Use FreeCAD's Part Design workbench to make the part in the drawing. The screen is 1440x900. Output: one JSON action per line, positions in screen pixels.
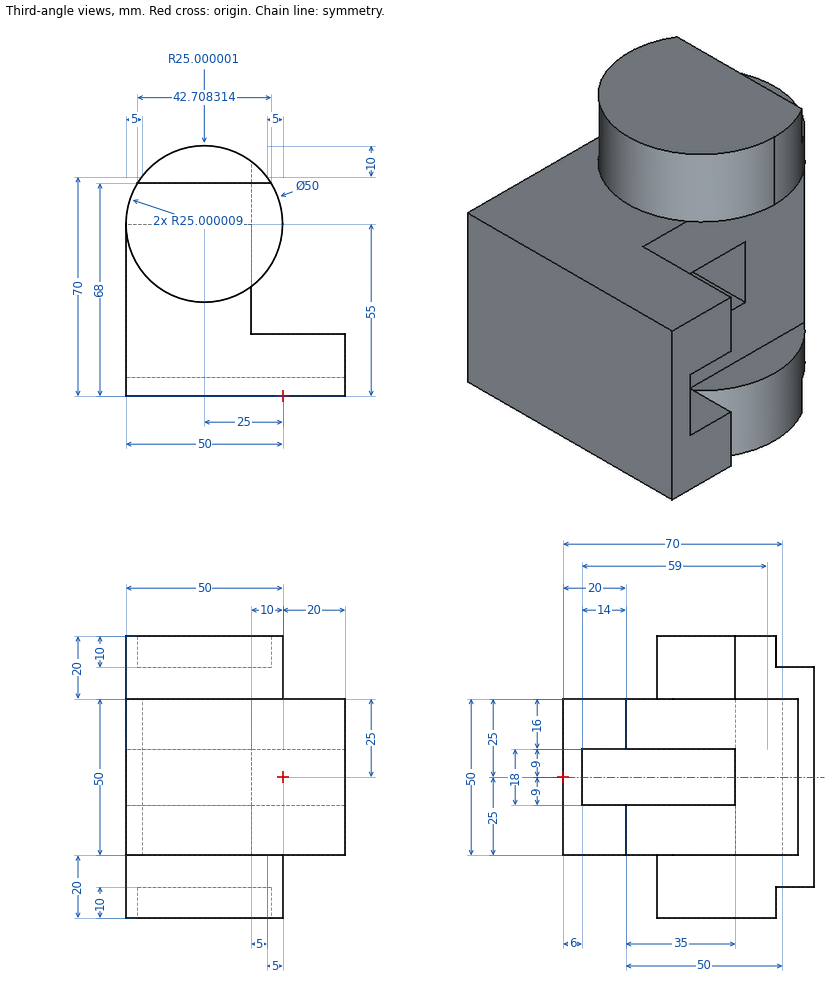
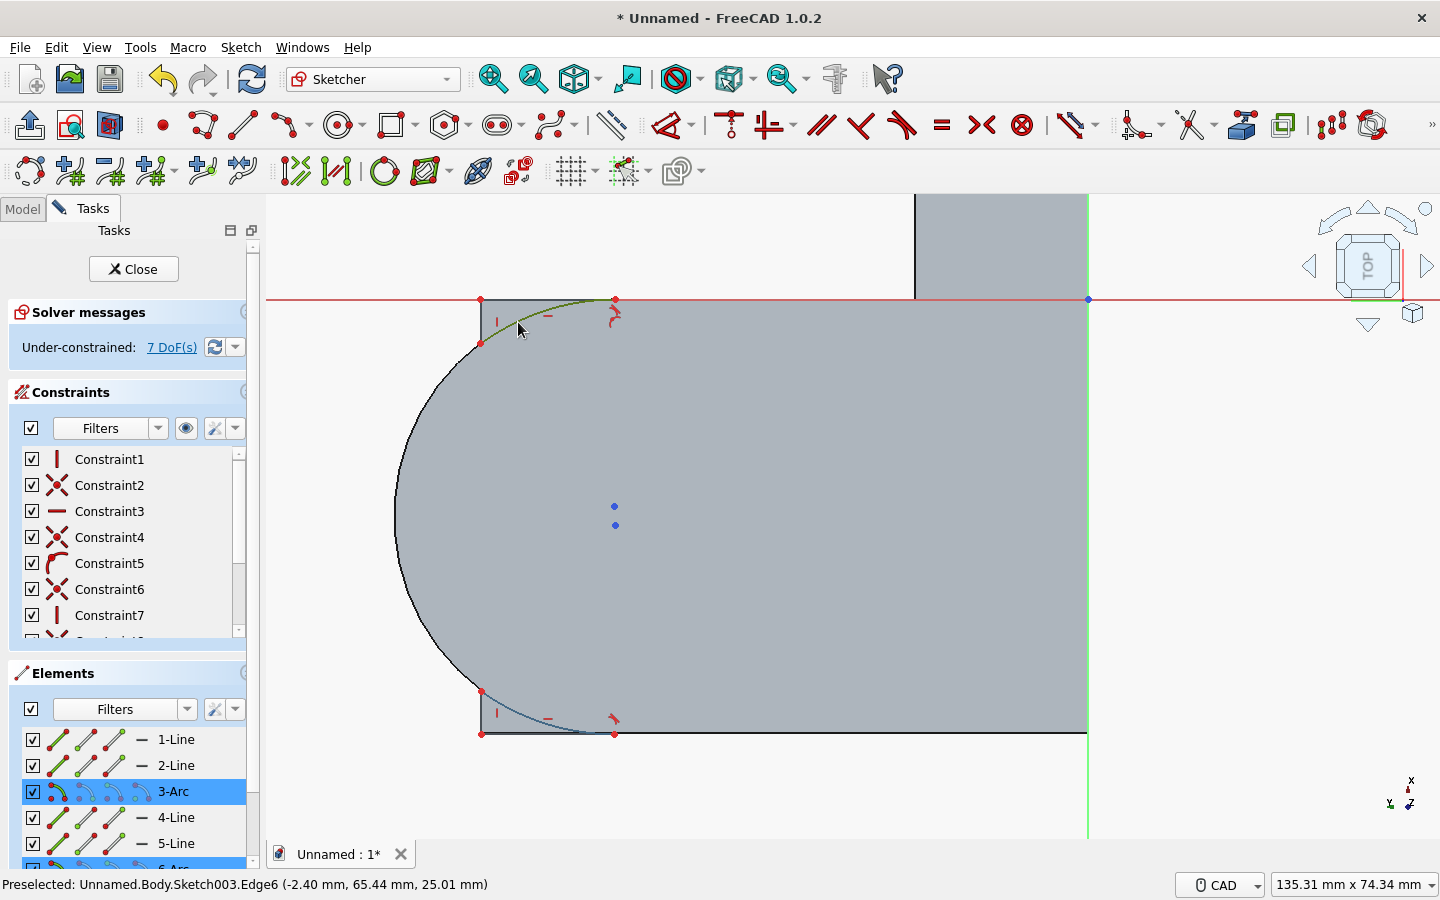
{"action": "left_click", "coordinate": [730, 126]}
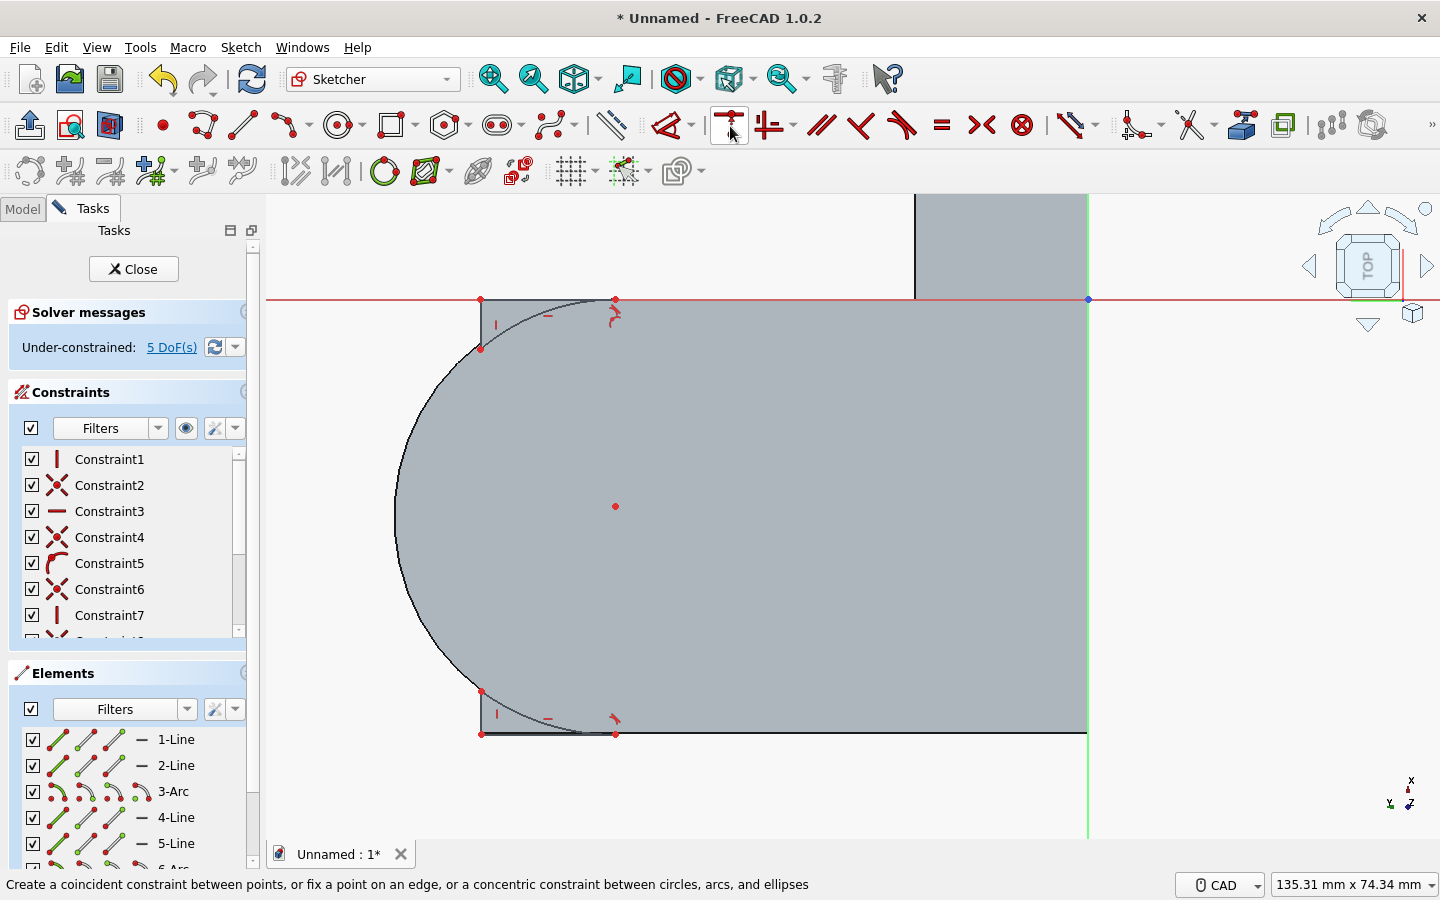
{"action": "left_click", "coordinate": [518, 713]}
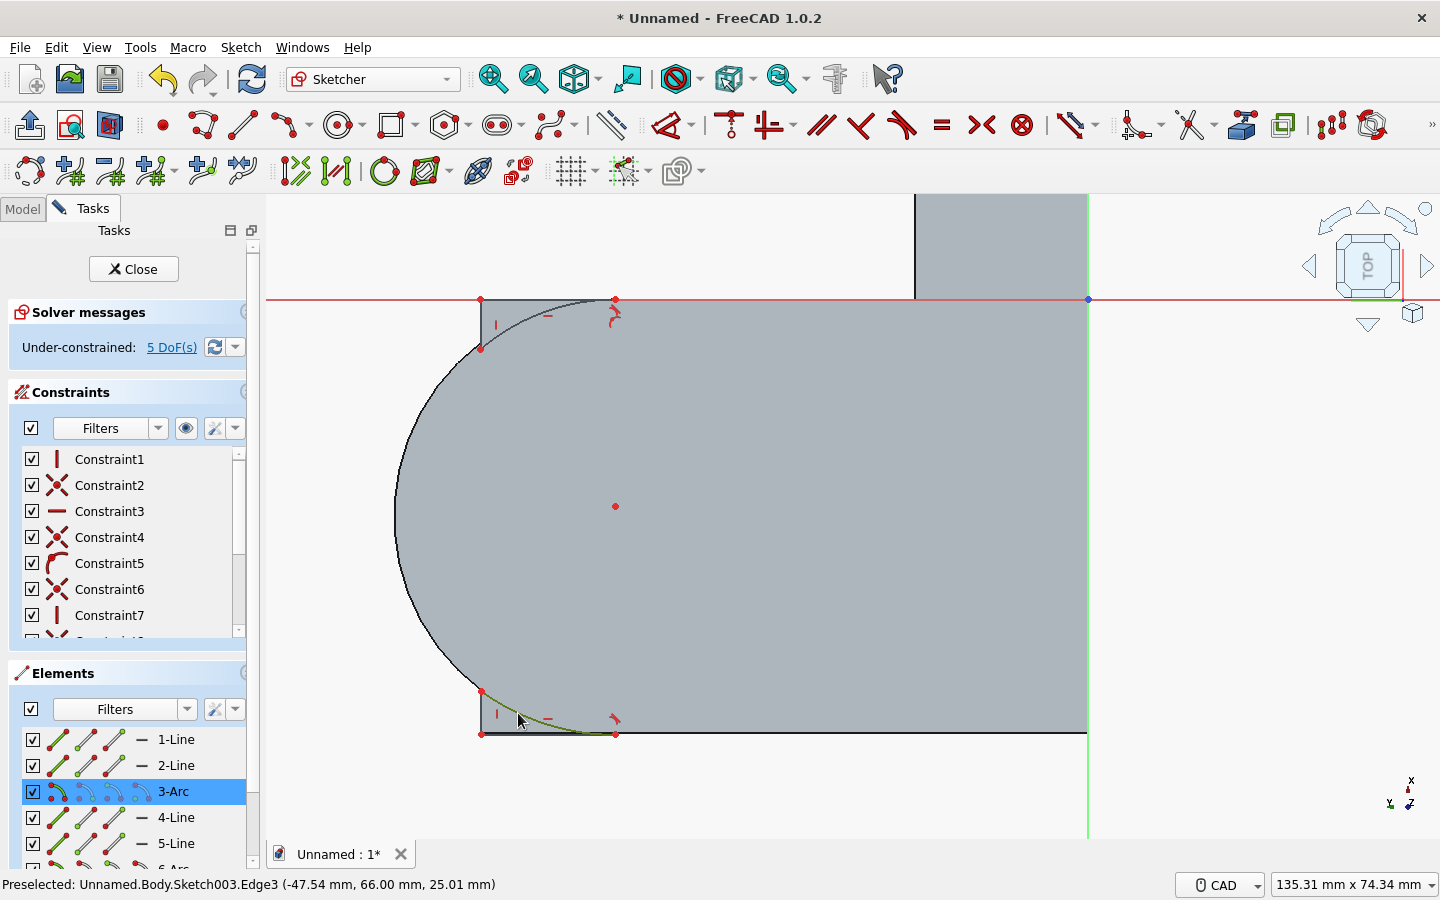
{"action": "left_click", "coordinate": [517, 324]}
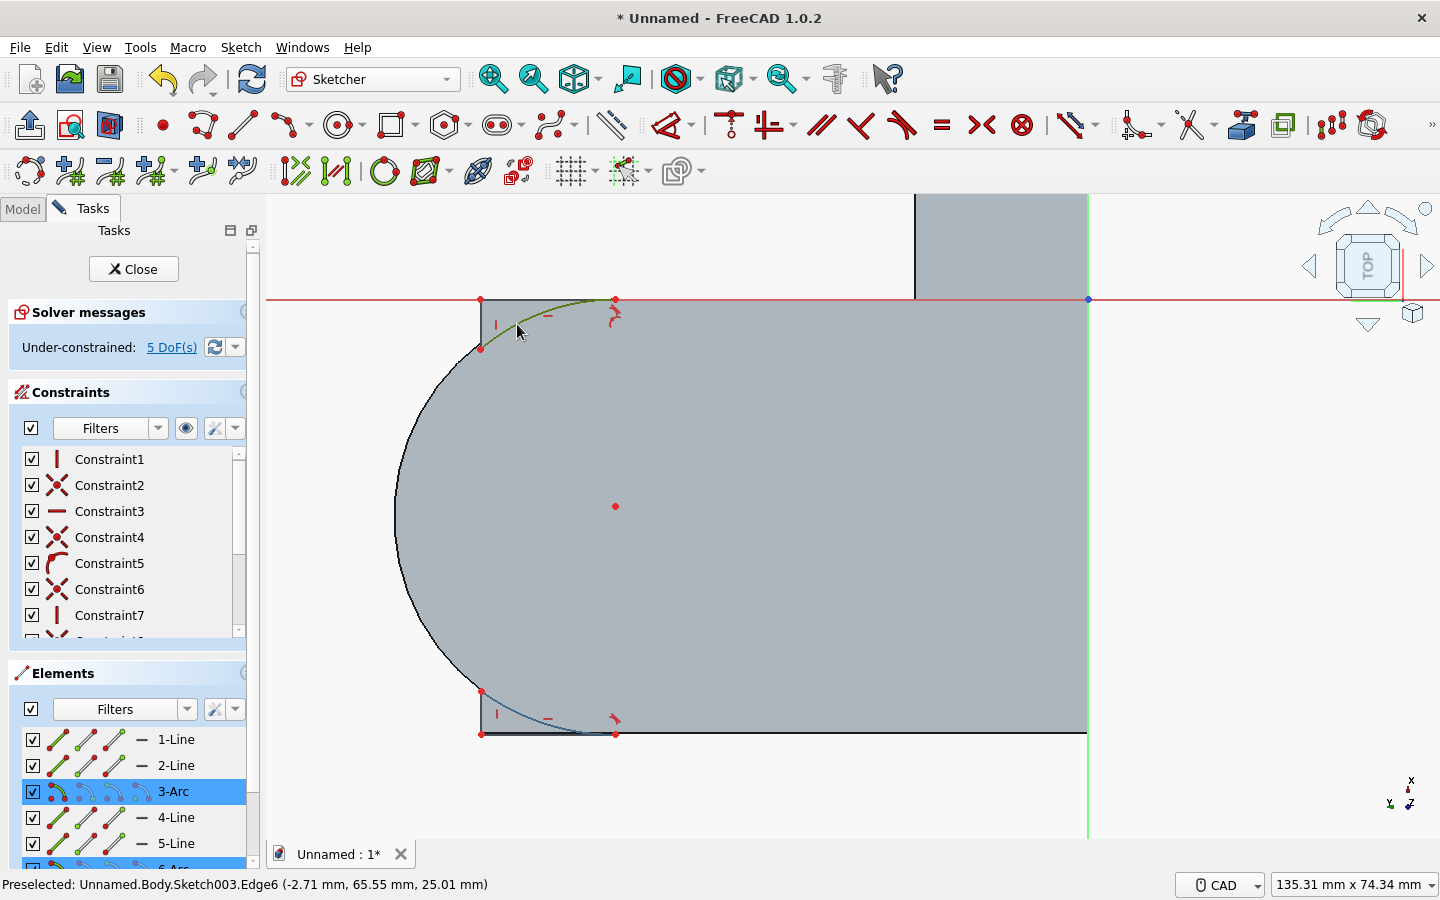
{"action": "left_click", "coordinate": [942, 126]}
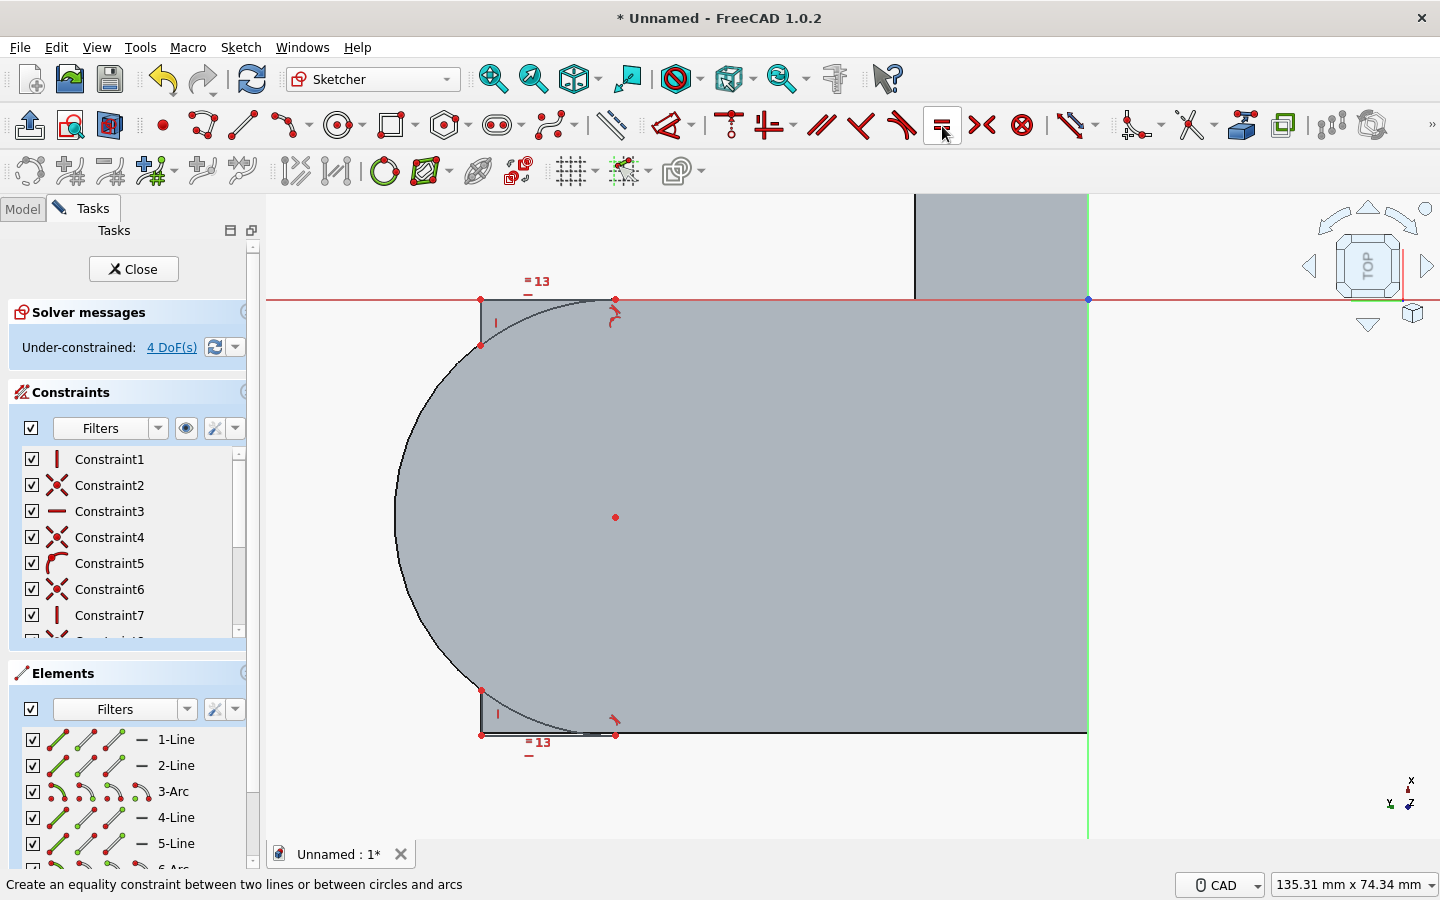
{"action": "left_click", "coordinate": [666, 126]}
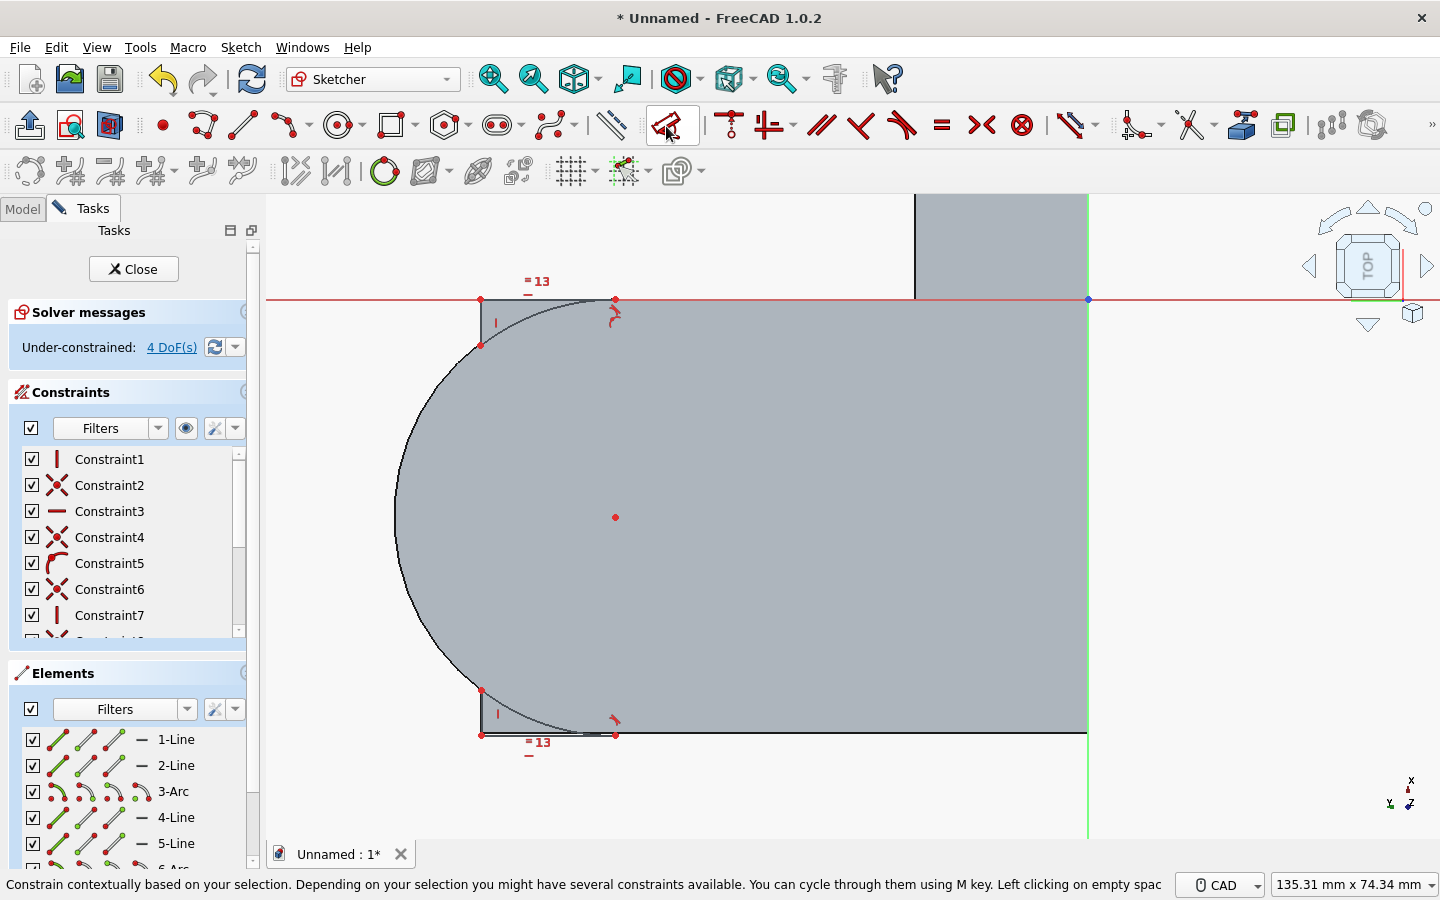
{"action": "left_click", "coordinate": [518, 713]}
{"action": "left_click", "coordinate": [410, 661]}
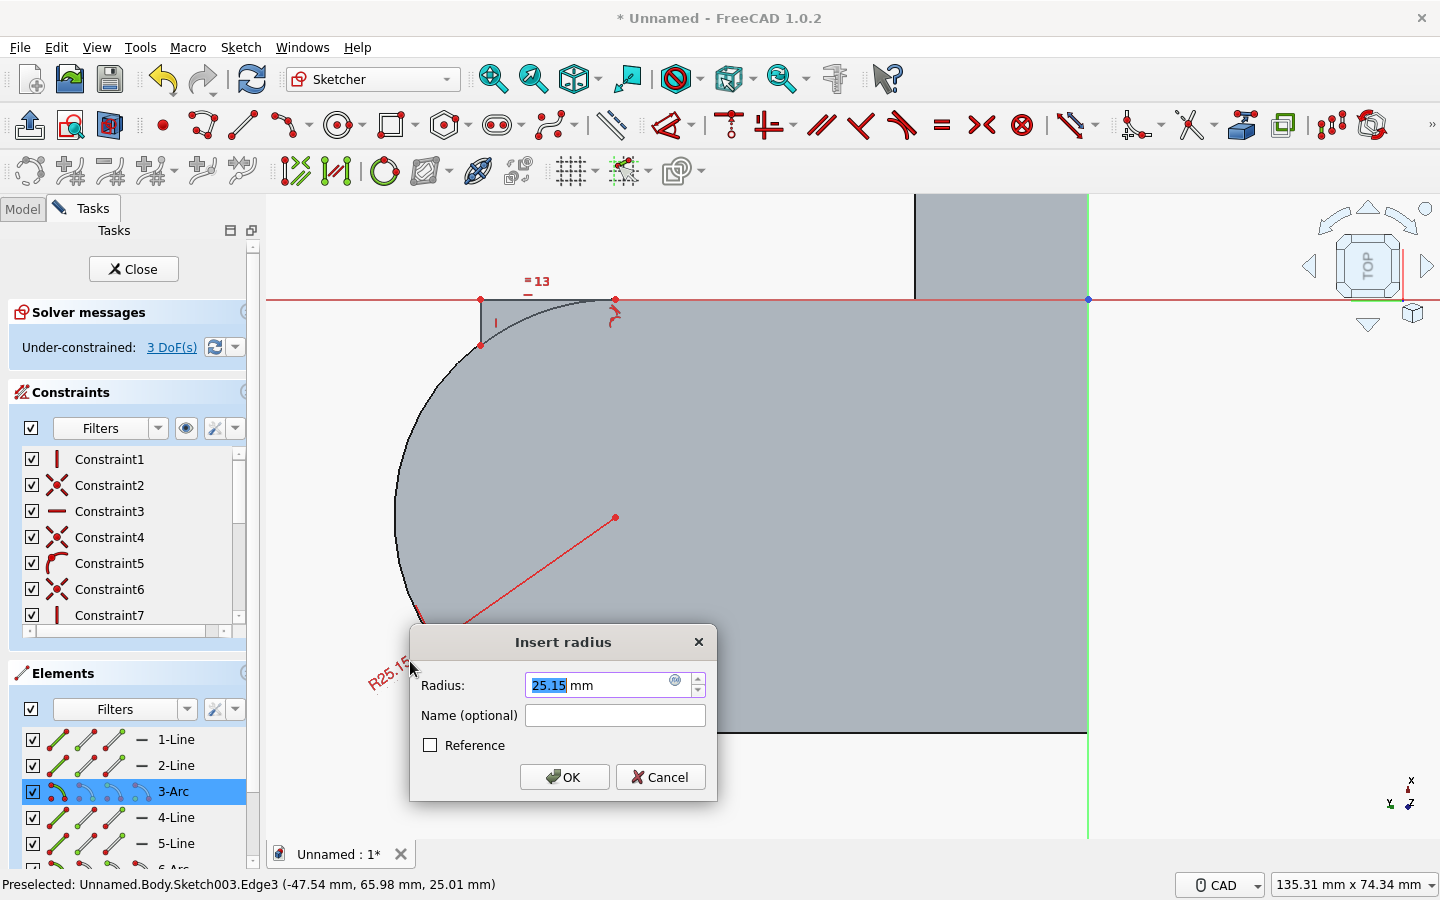
{"action": "type", "text": "25.000009"}
{"action": "key", "text": "Return"}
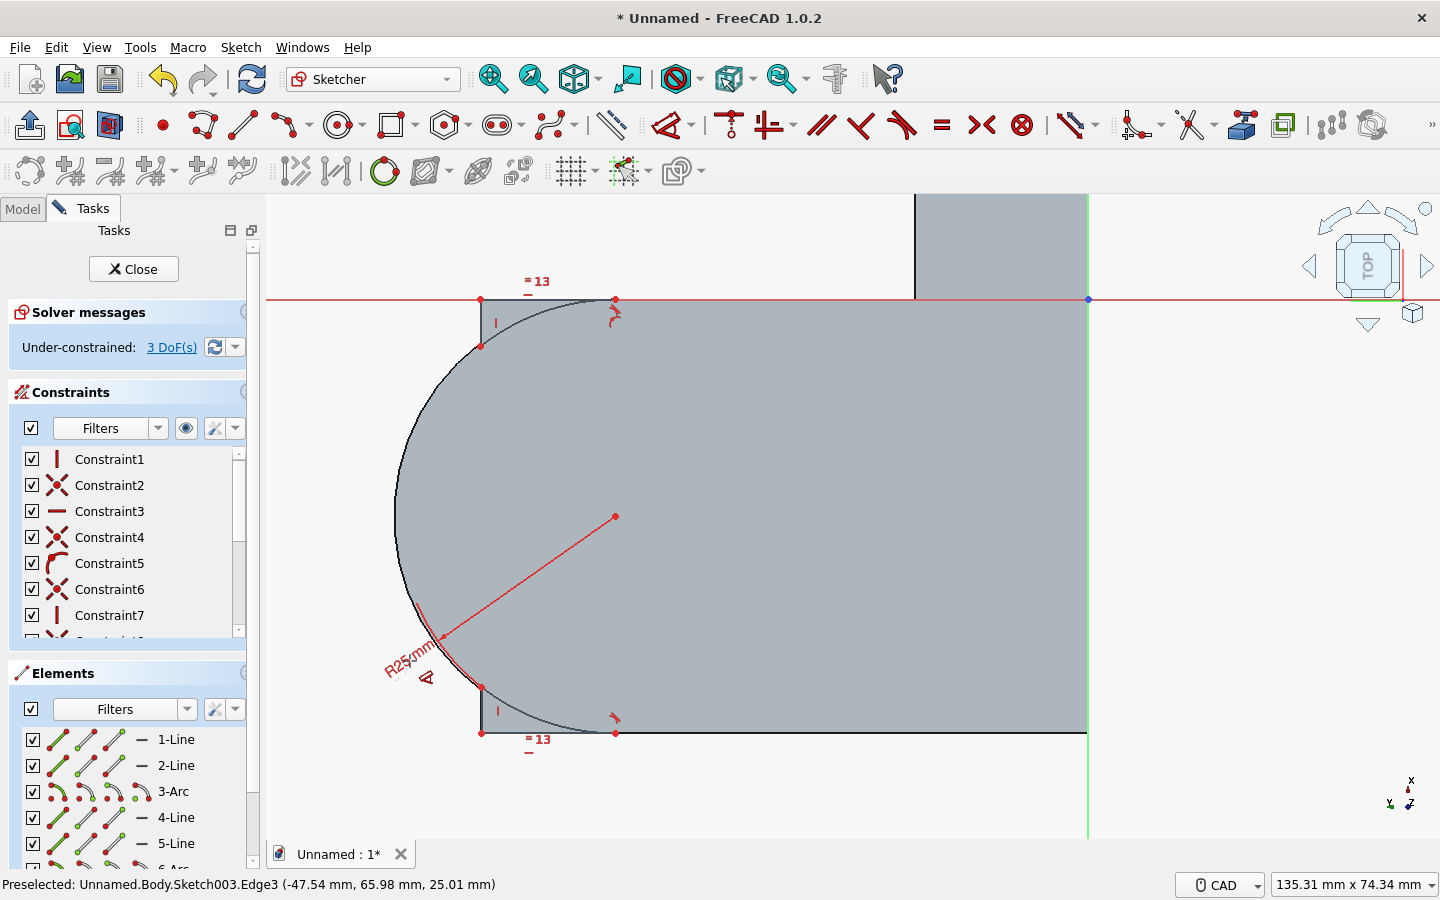
{"action": "scroll", "coordinate": [482, 701], "scroll_direction": "up", "scroll_amount": 2}